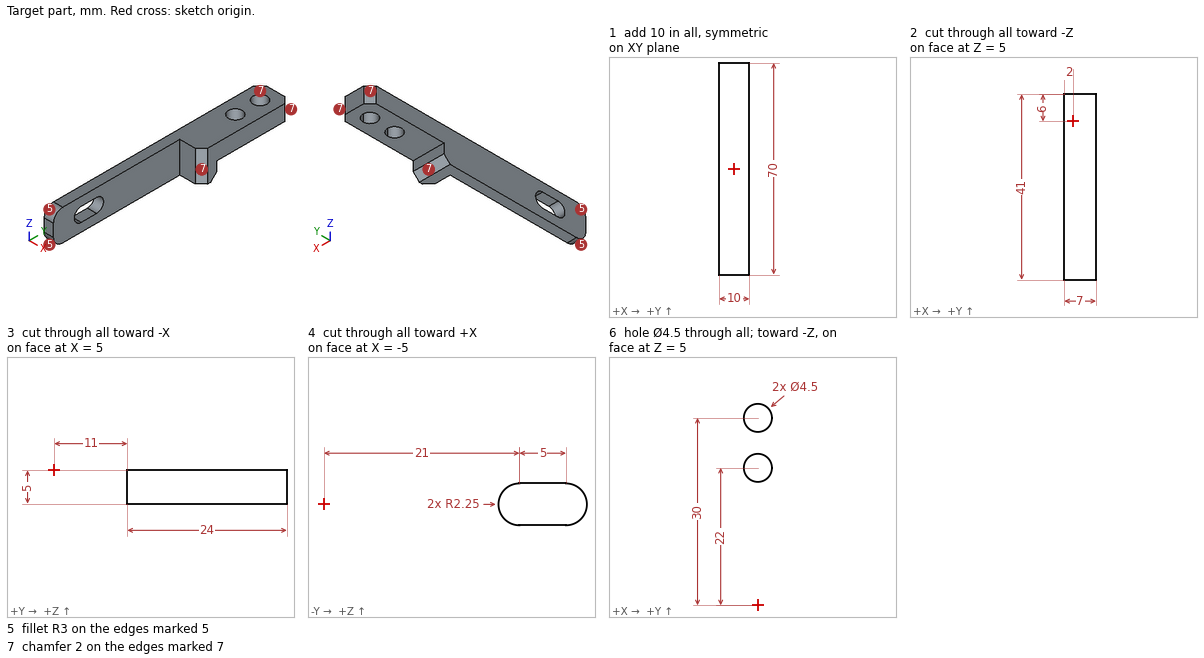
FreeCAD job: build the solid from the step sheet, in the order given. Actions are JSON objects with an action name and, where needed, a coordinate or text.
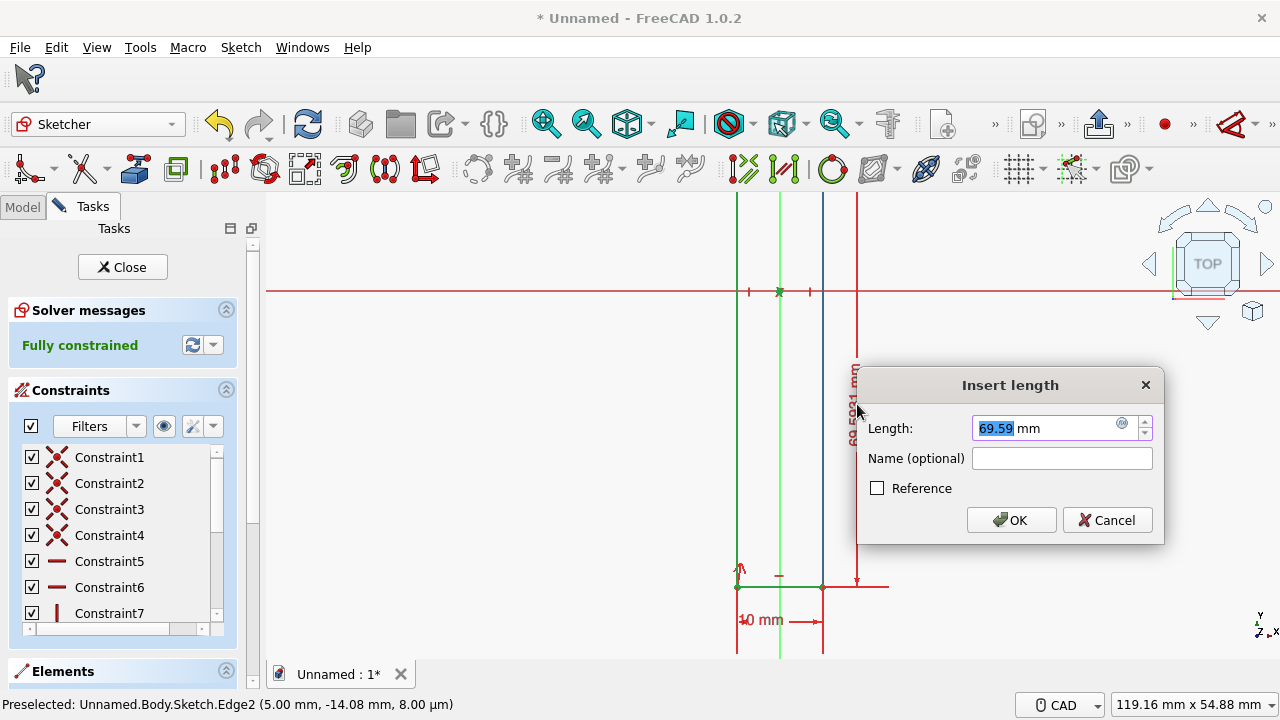
{"action": "type", "text": "70"}
{"action": "key", "text": "Return"}
{"action": "key", "text": "Escape"}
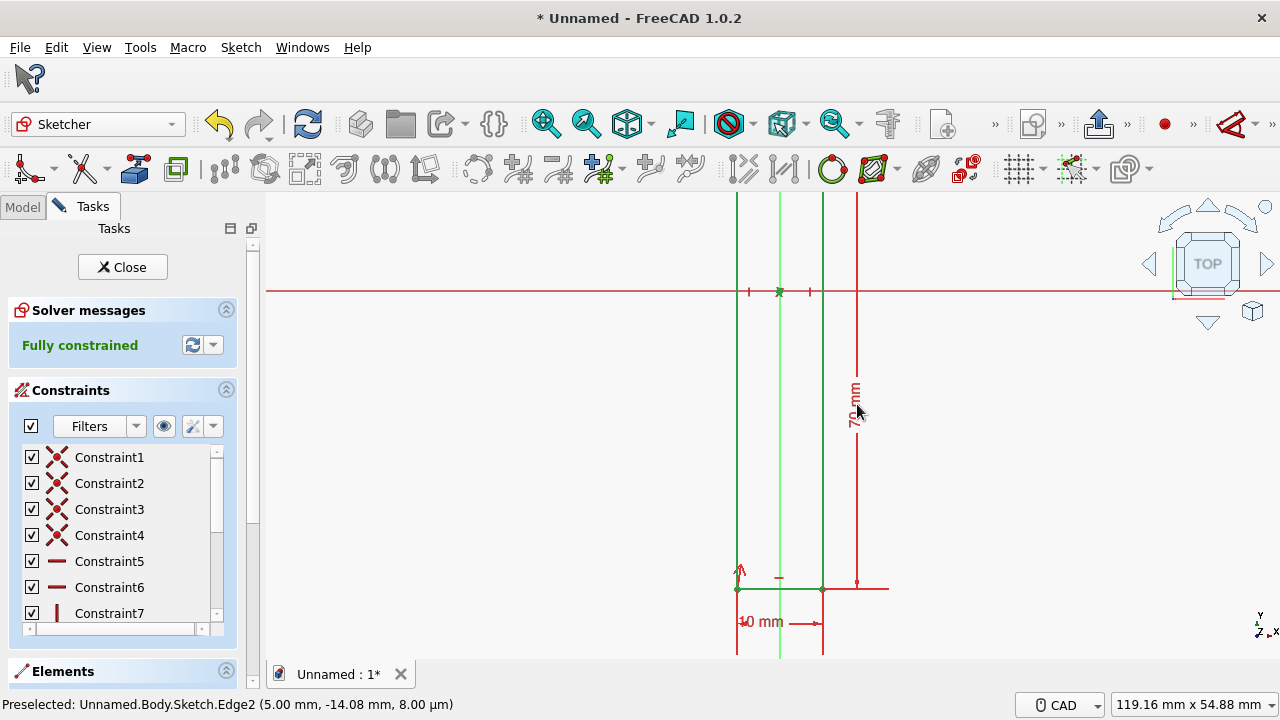
{"action": "left_click", "coordinate": [123, 267]}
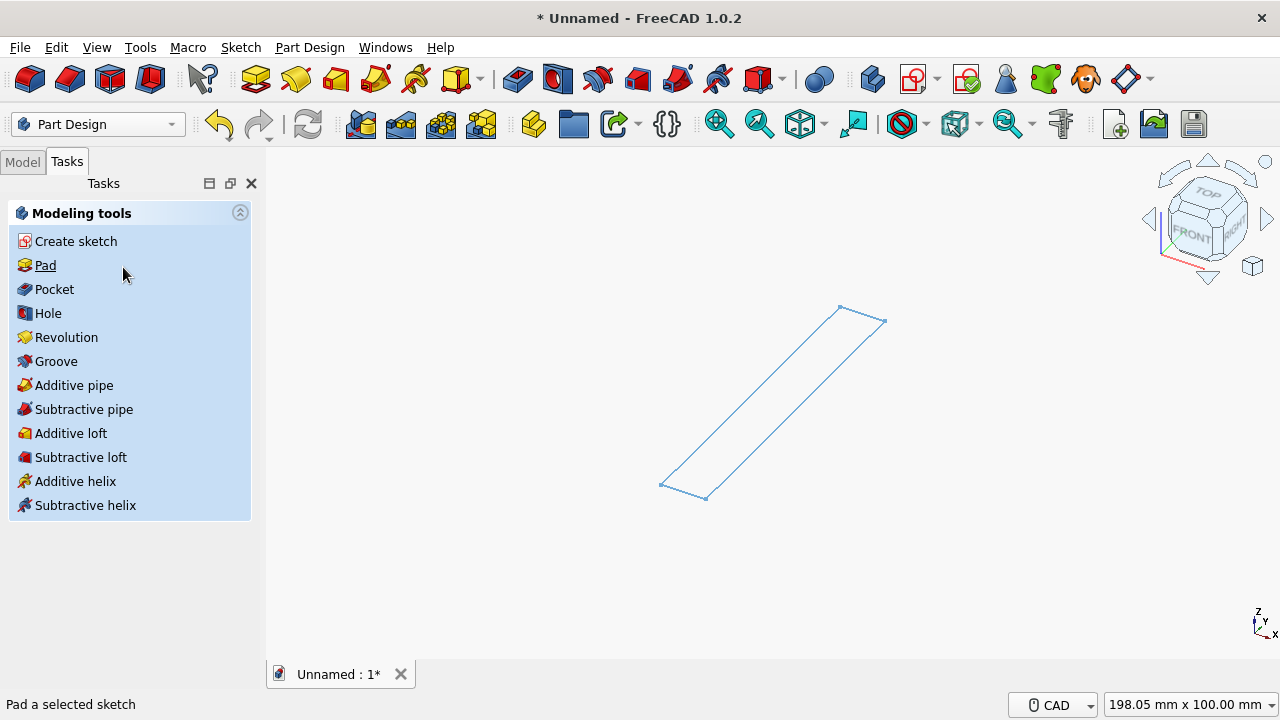
{"action": "left_click", "coordinate": [256, 80]}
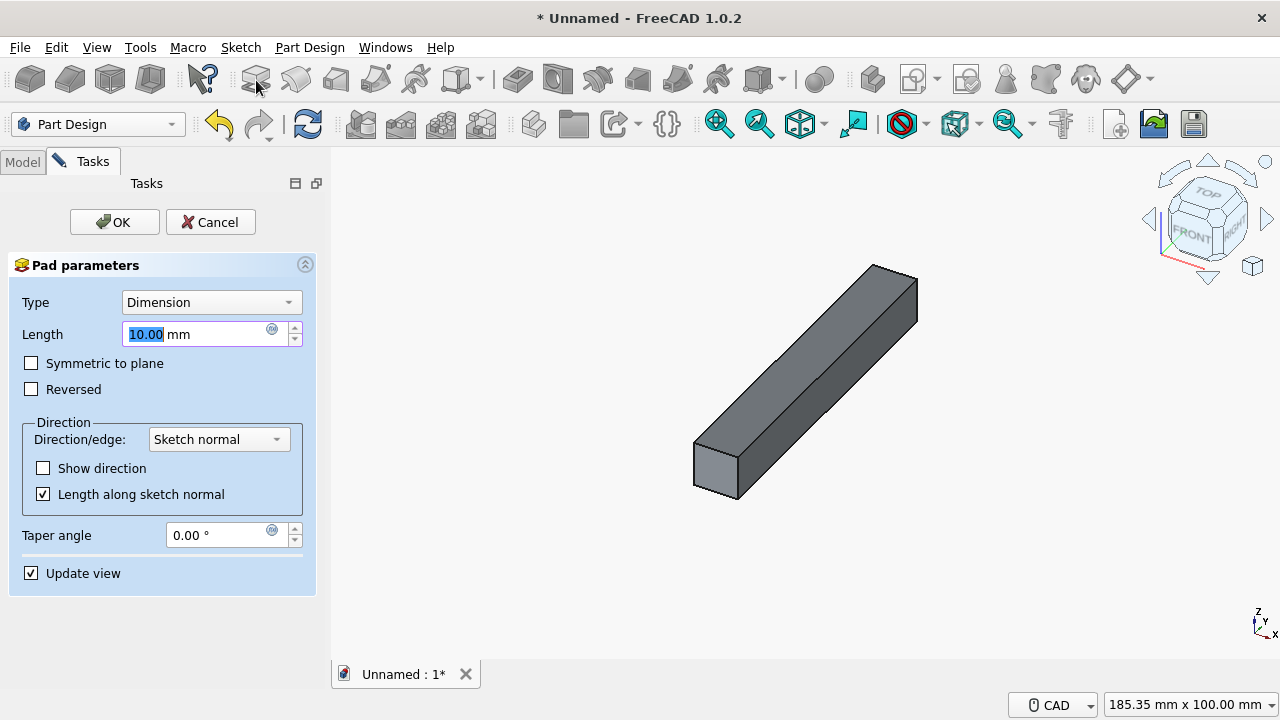
{"action": "type", "text": "10"}
{"action": "key", "text": "Tab"}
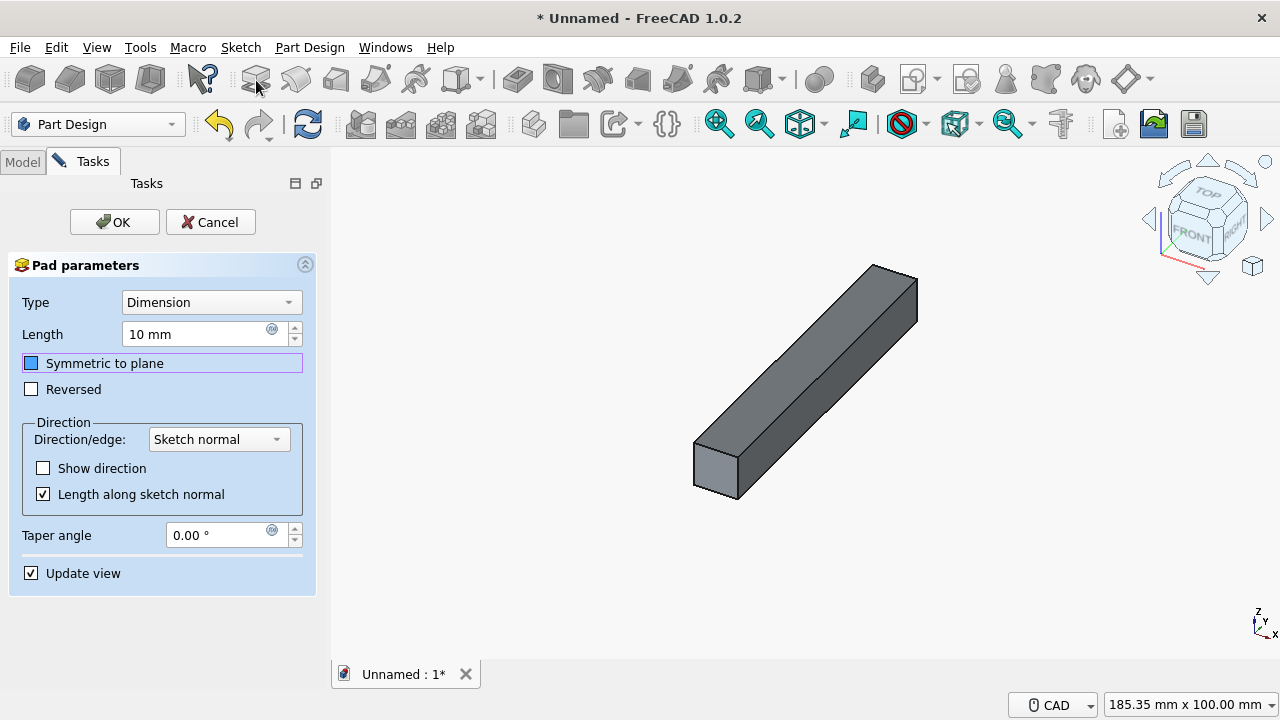
{"action": "left_click", "coordinate": [30, 363]}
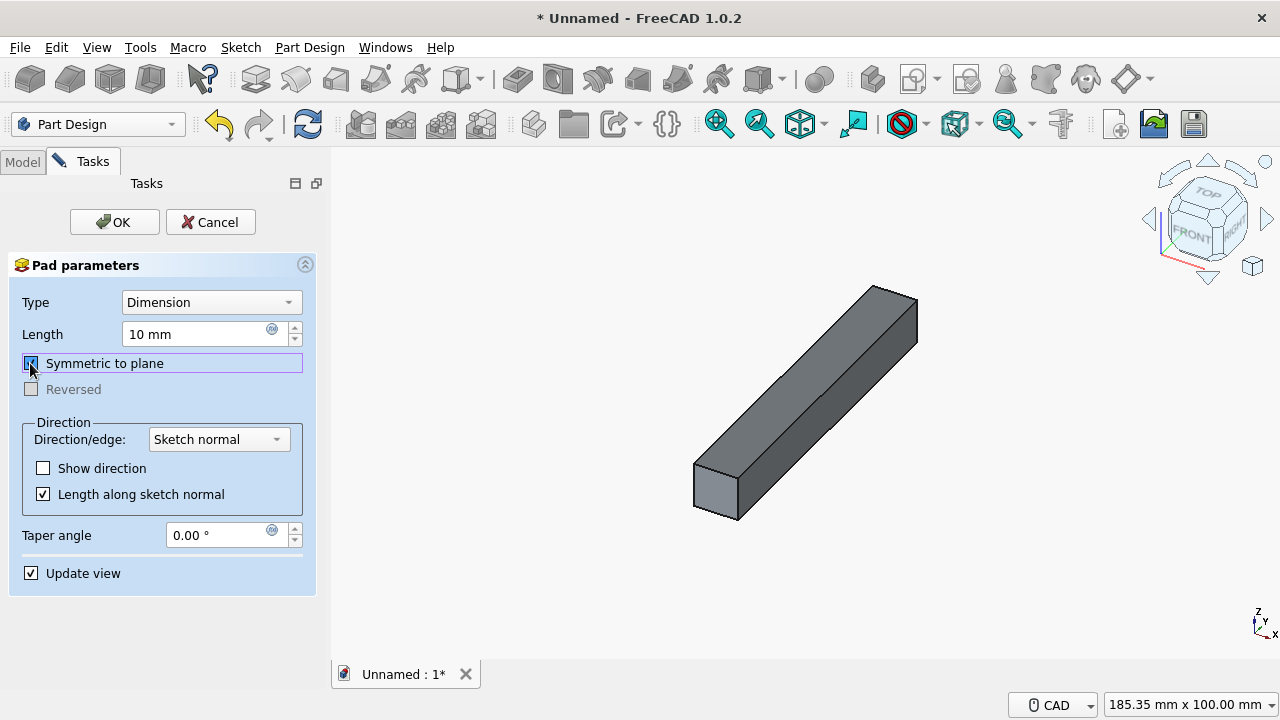
{"action": "left_click", "coordinate": [115, 222]}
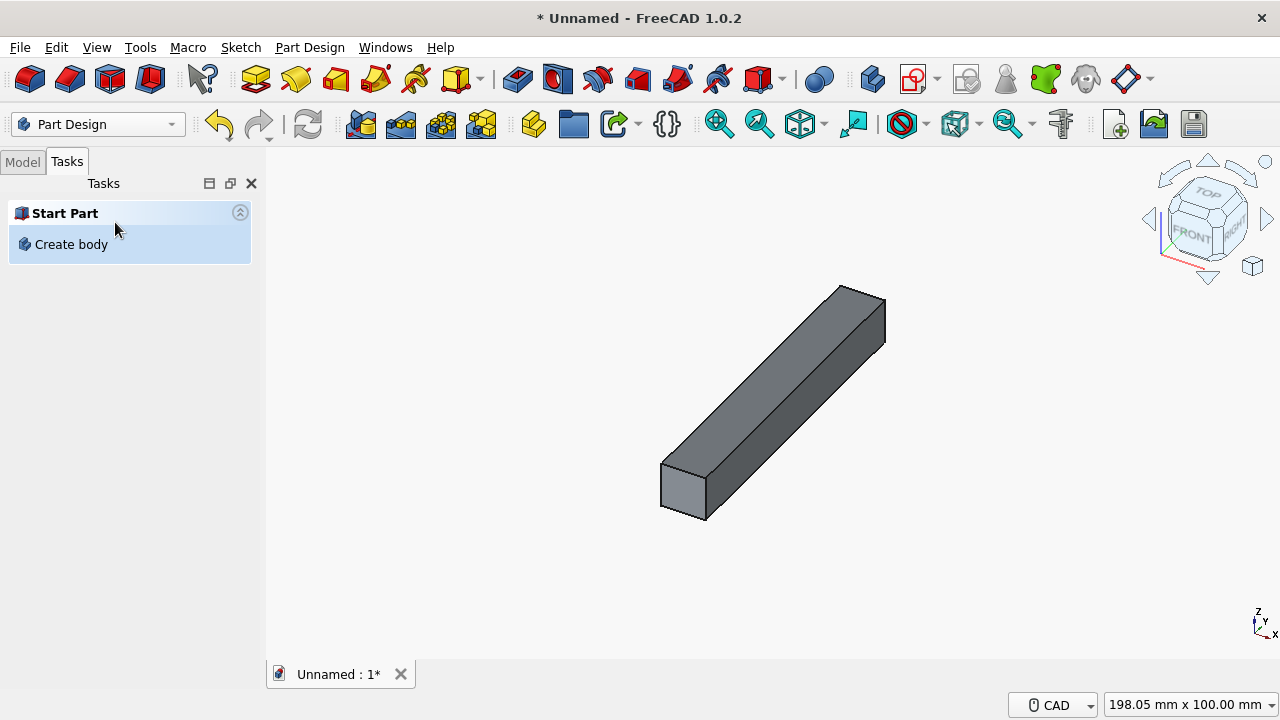
{"action": "left_click", "coordinate": [850, 305]}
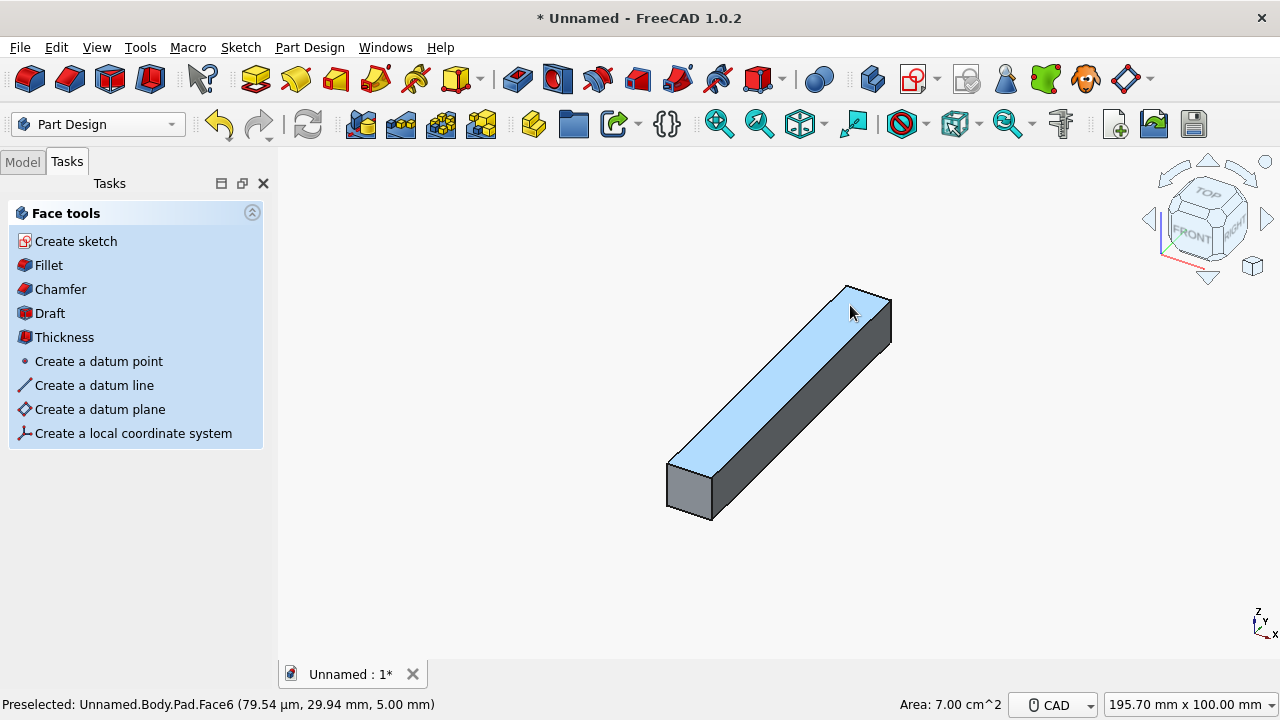
{"action": "left_click", "coordinate": [914, 80]}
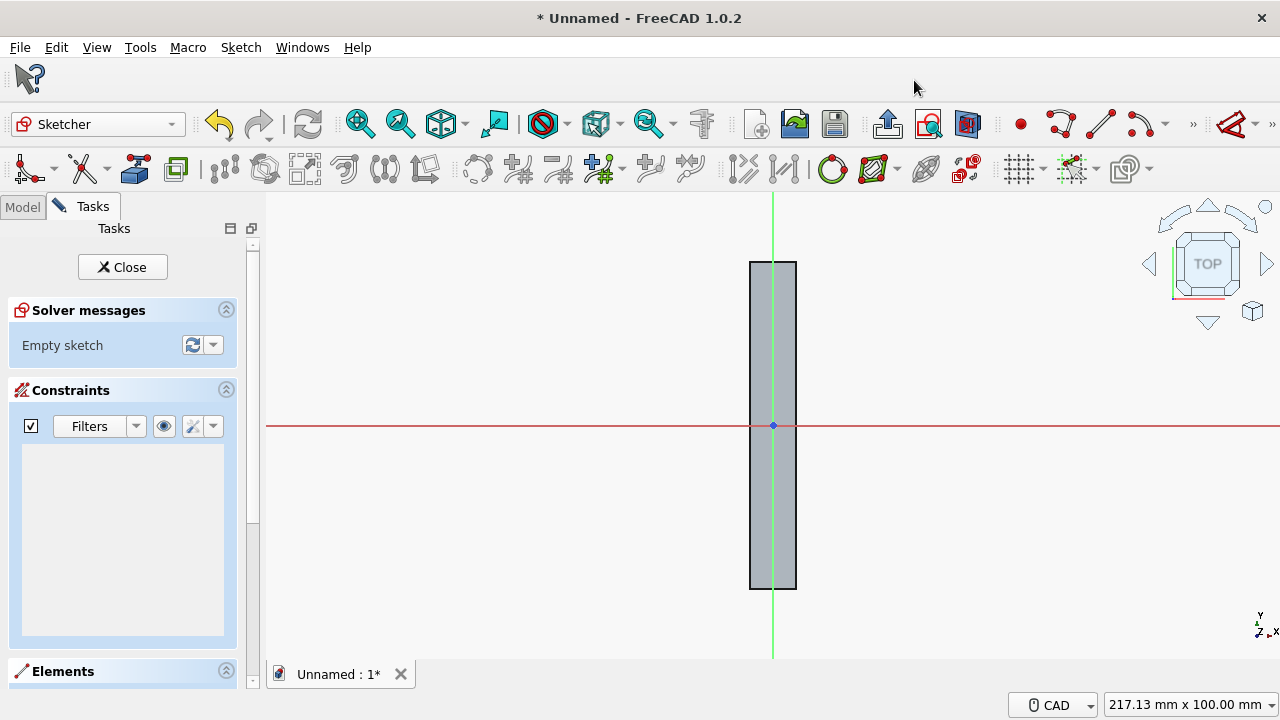
{"action": "scroll", "coordinate": [934, 631], "scroll_direction": "up", "scroll_amount": 2}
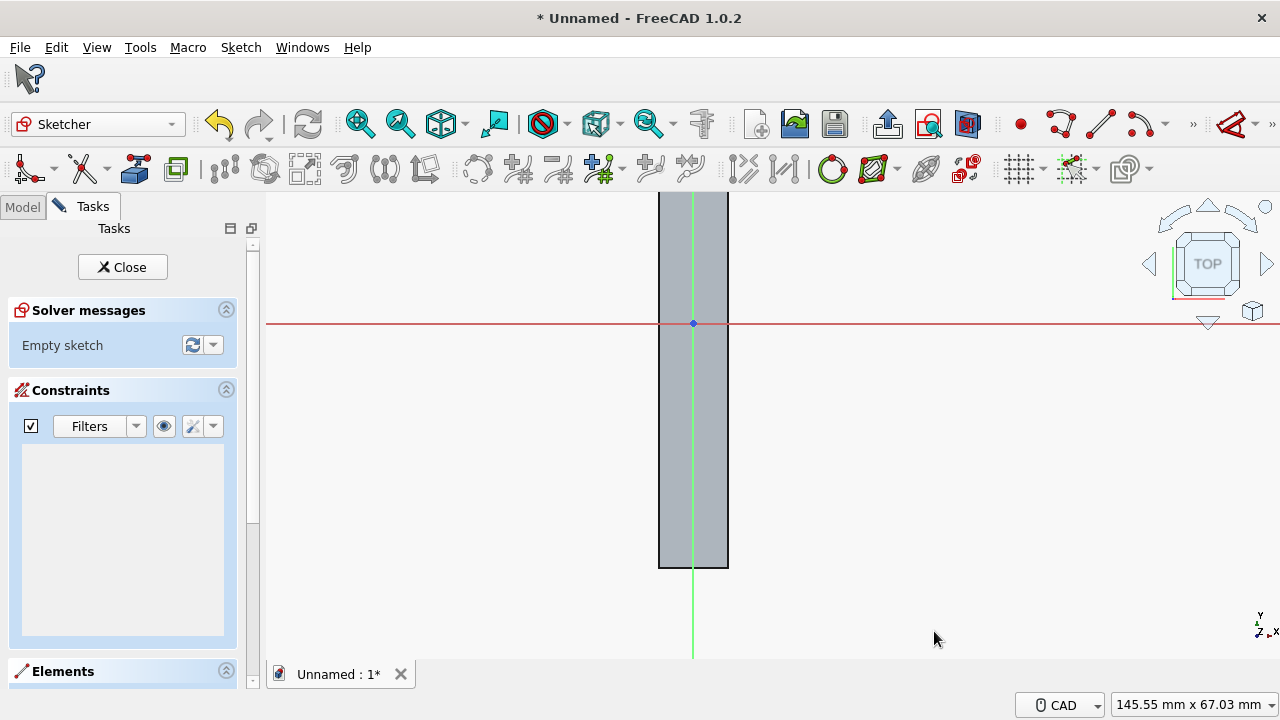
{"action": "key", "text": "g r"}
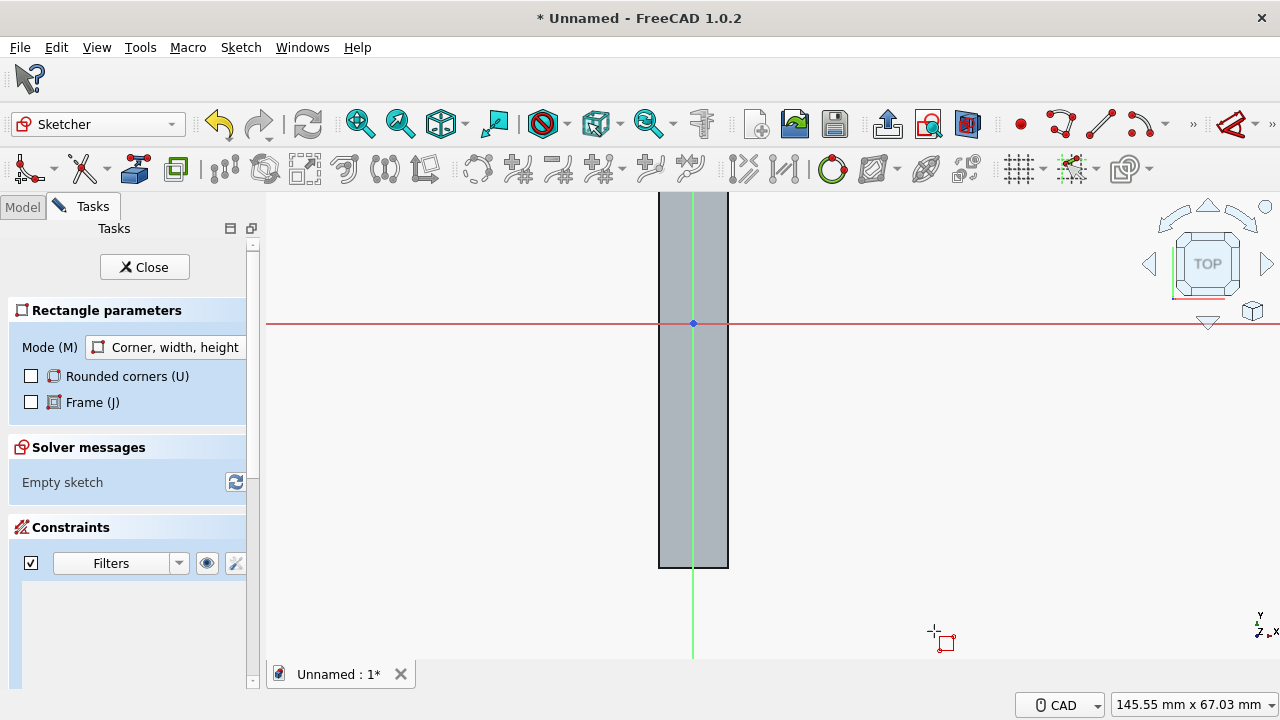
{"action": "left_click", "coordinate": [680, 282]}
{"action": "left_click", "coordinate": [728, 568]}
{"action": "key", "text": "Escape"}